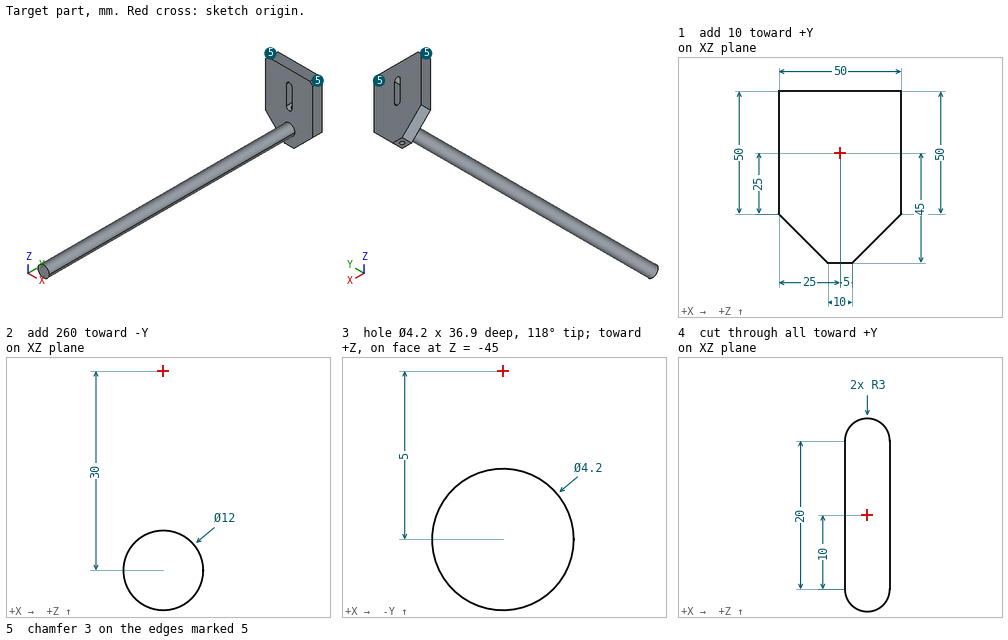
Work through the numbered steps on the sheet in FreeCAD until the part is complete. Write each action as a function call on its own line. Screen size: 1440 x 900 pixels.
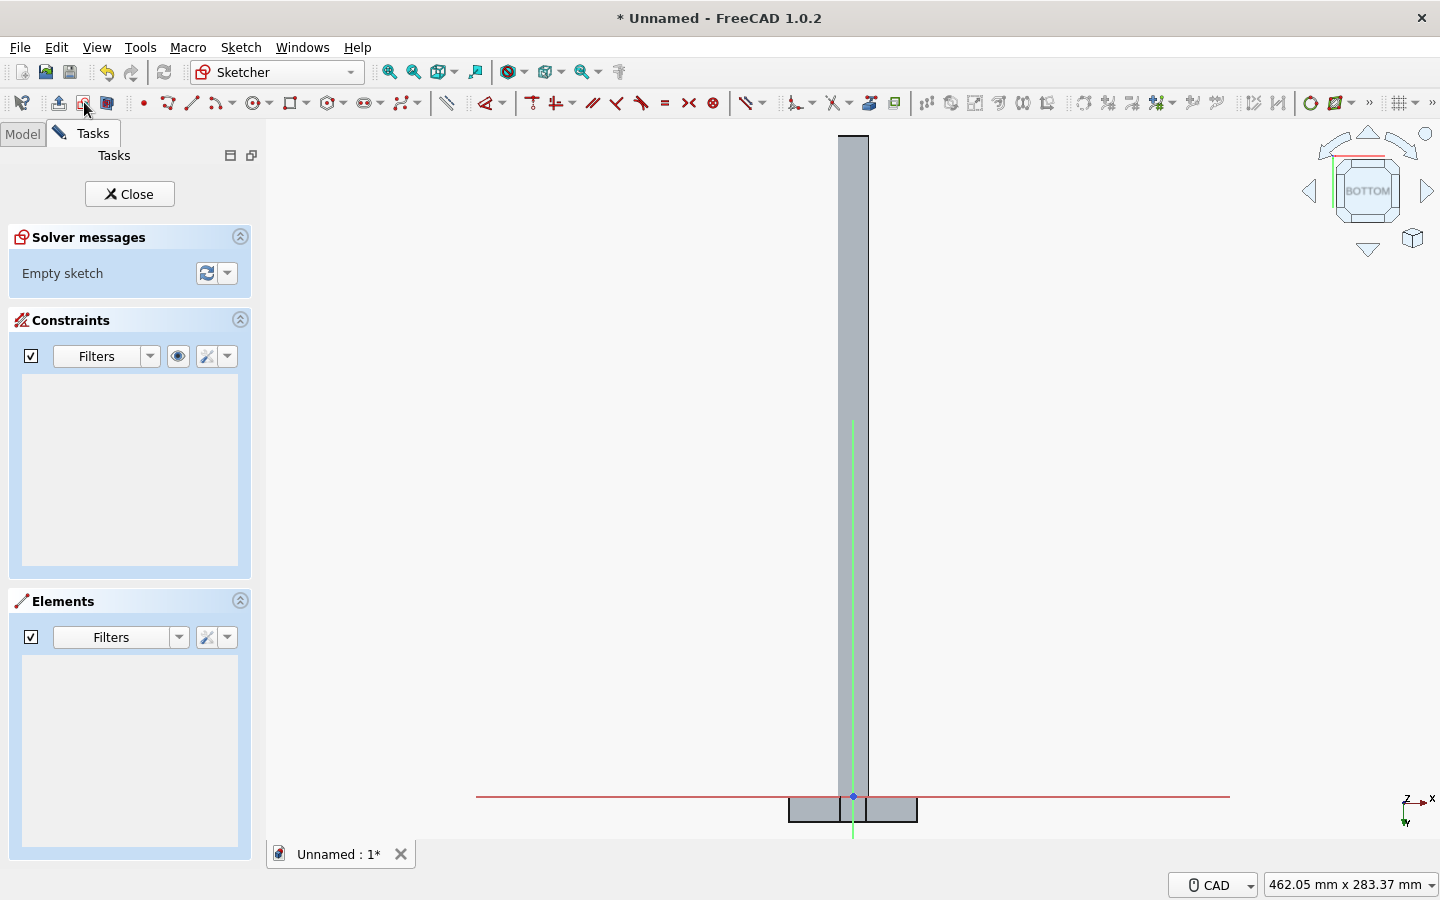
scroll(784, 479, down, 5)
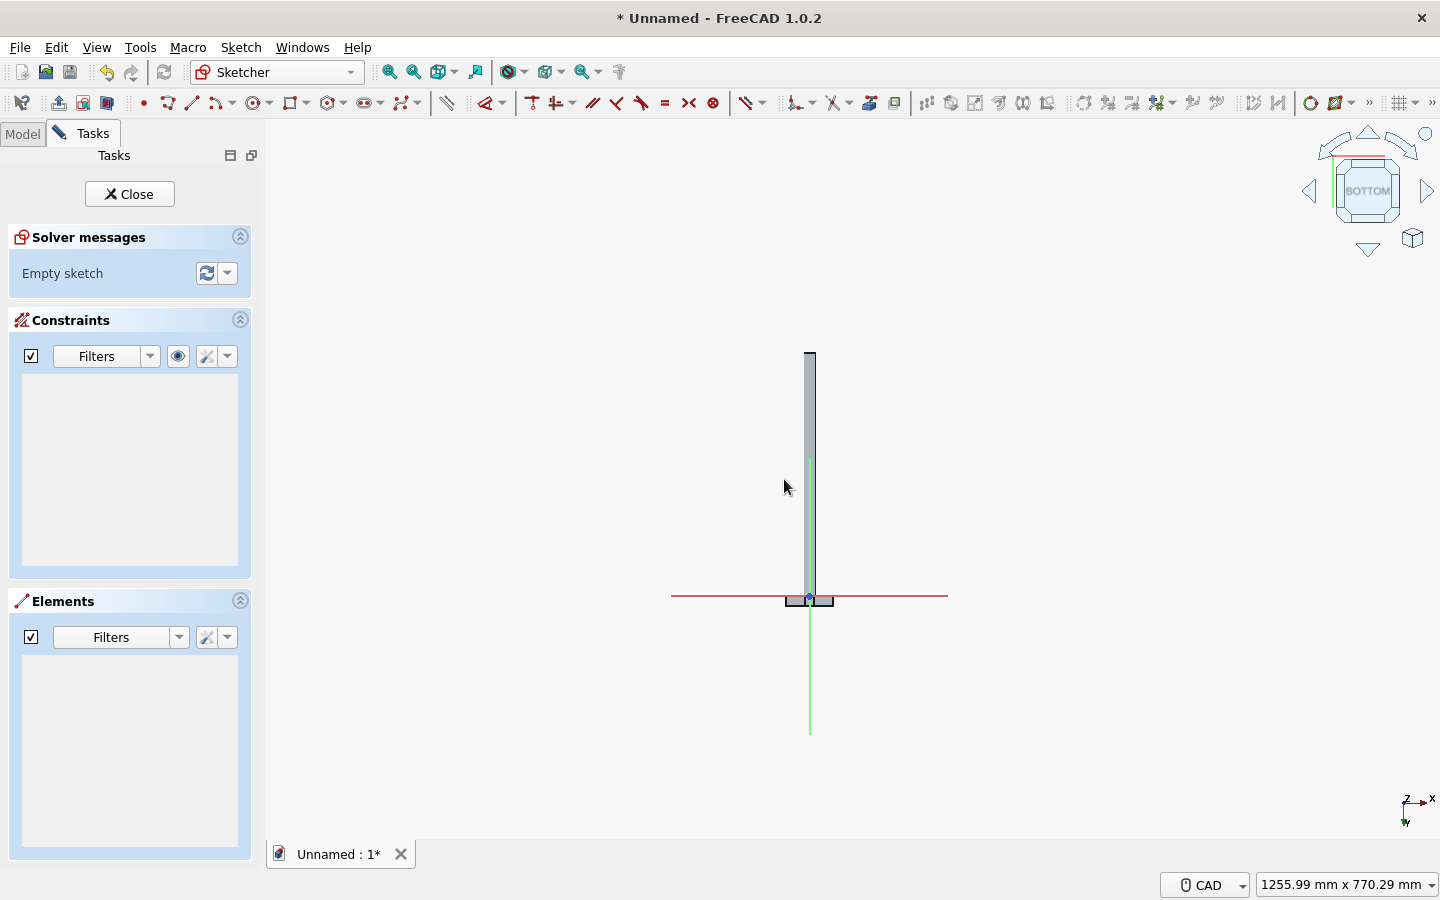
scroll(811, 606, up, 15)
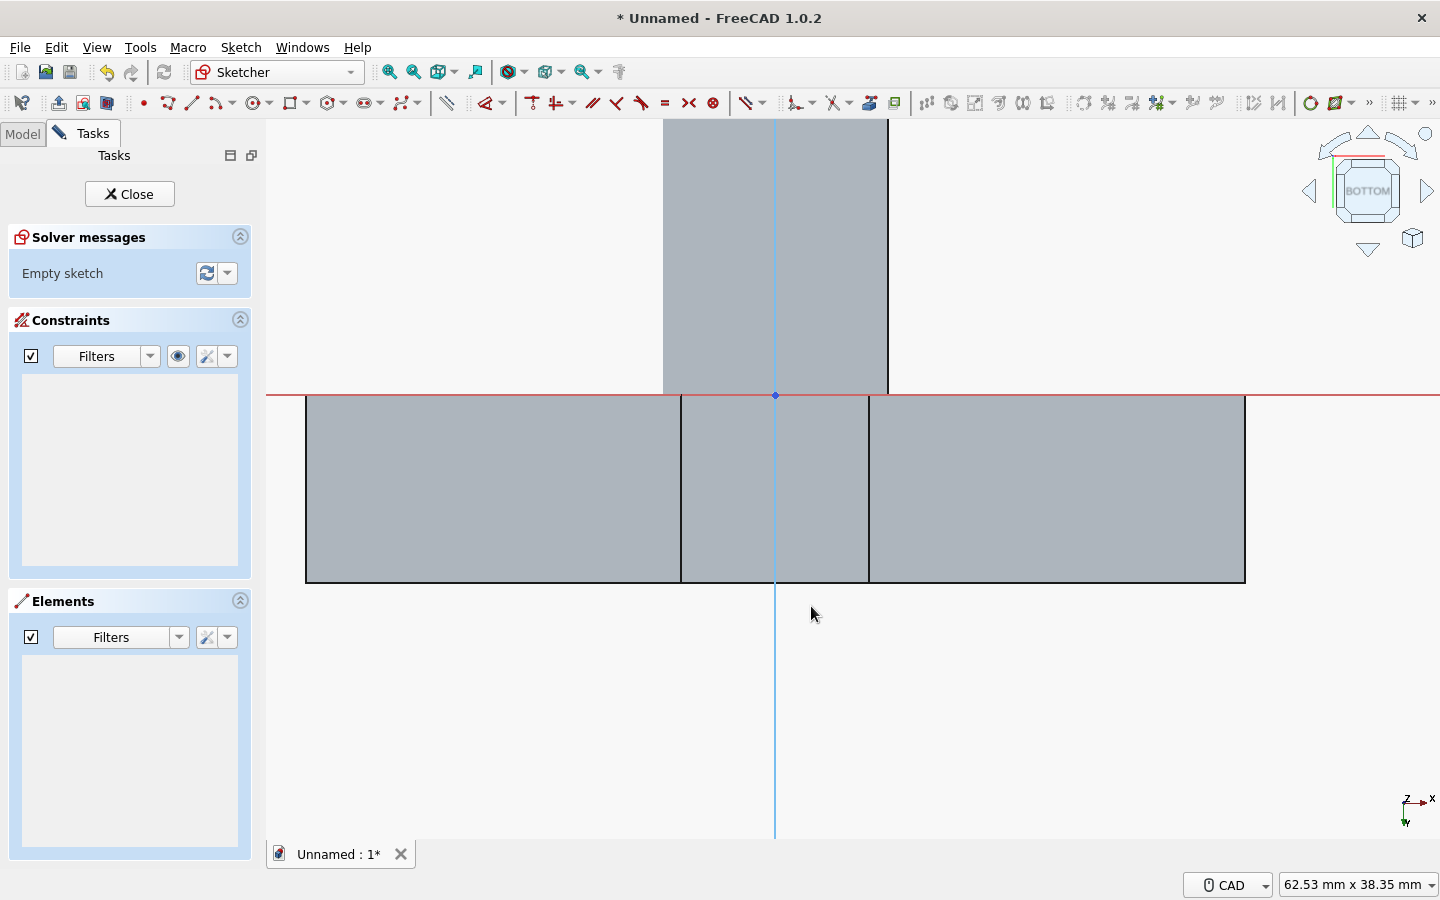
scroll(771, 455, up, 6)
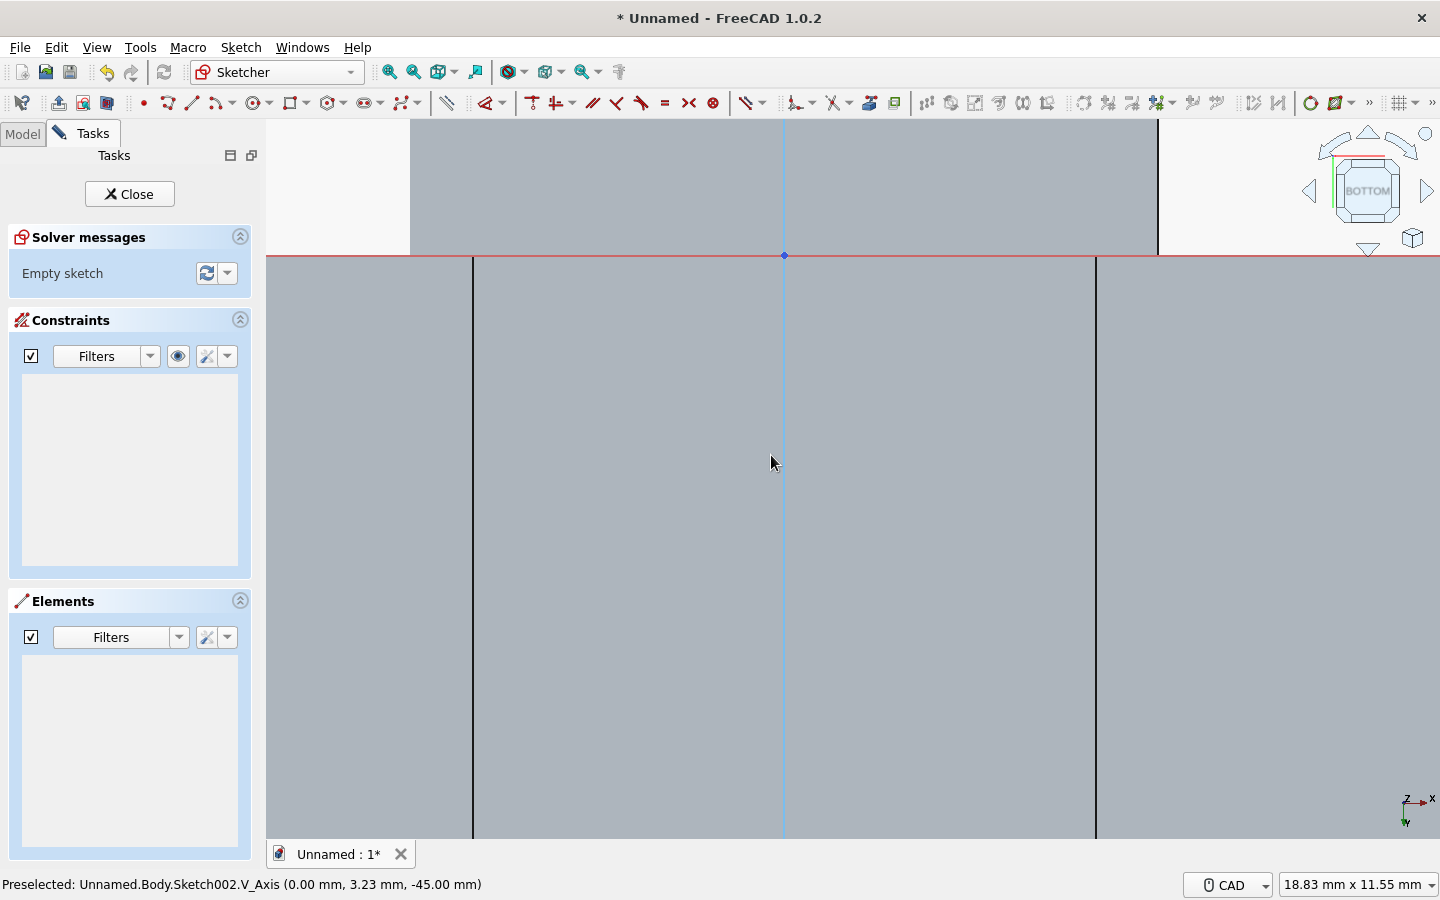
click(254, 104)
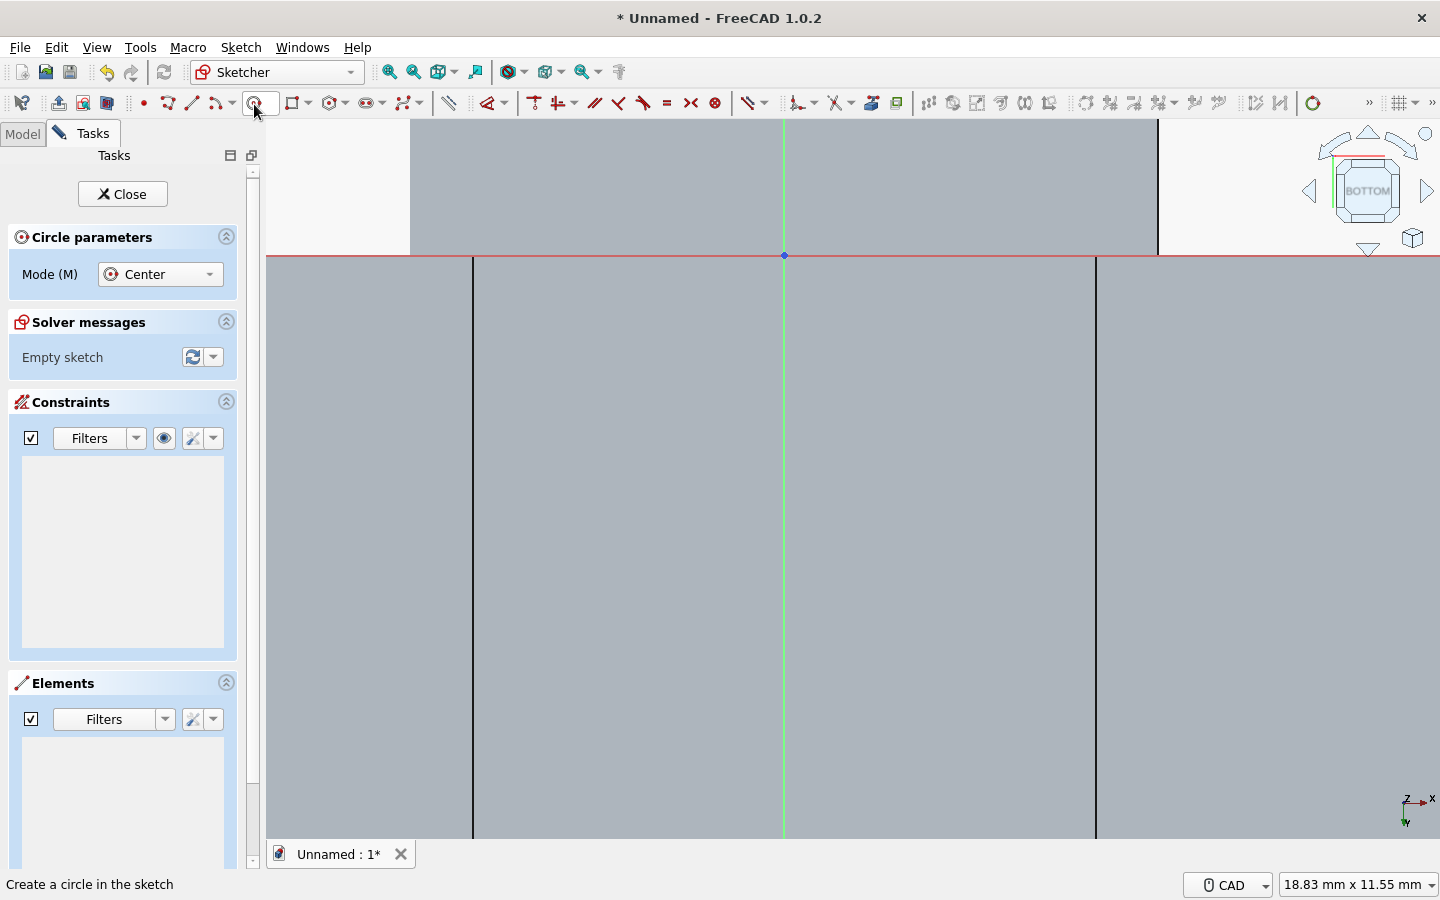
click(784, 568)
move(877, 475)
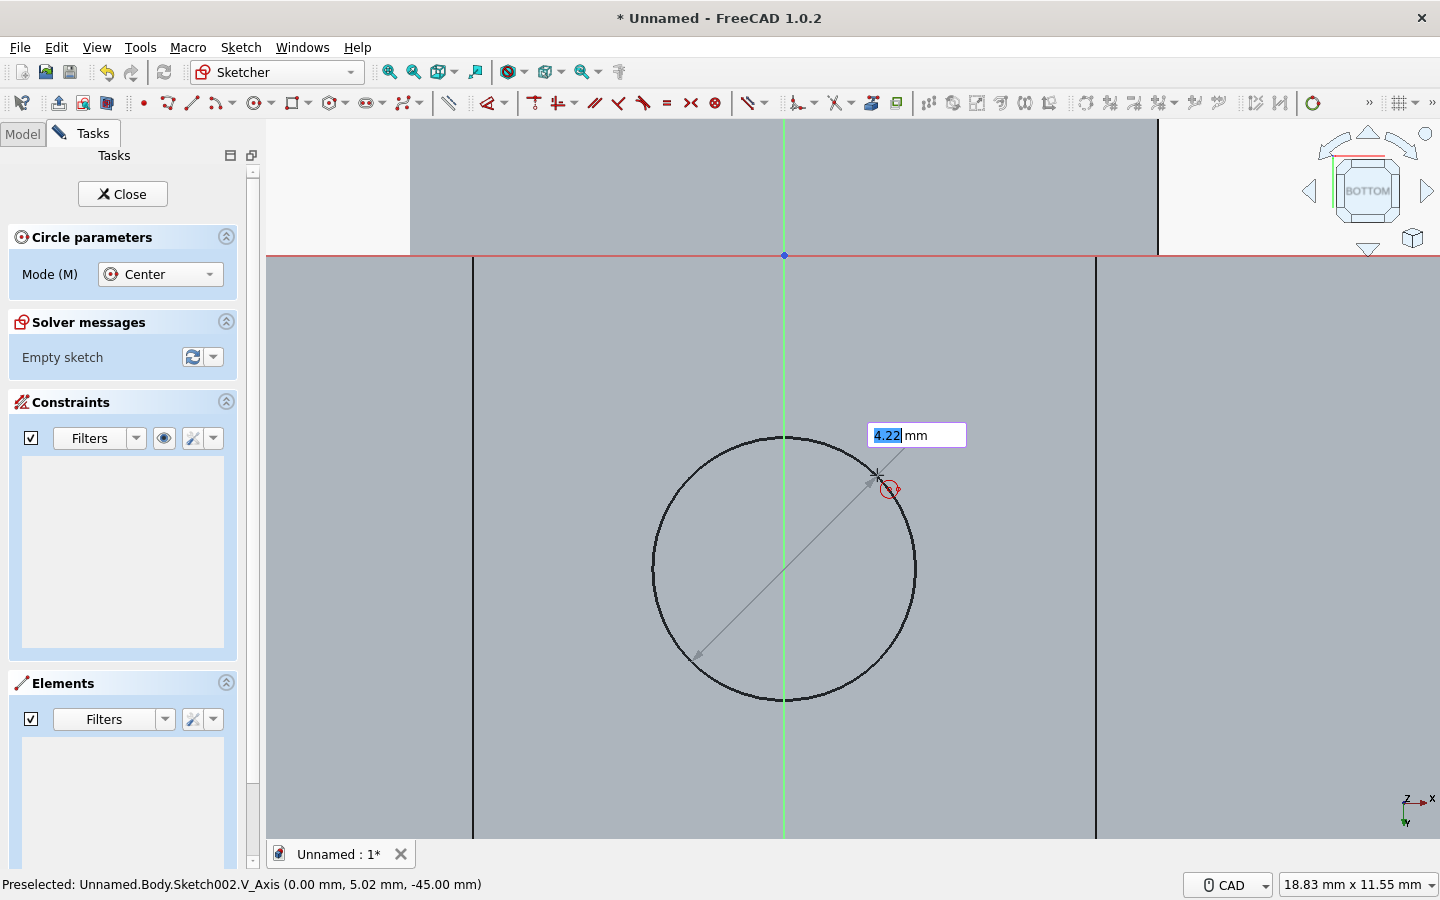
text(4.2)
key(Return)
key(Escape)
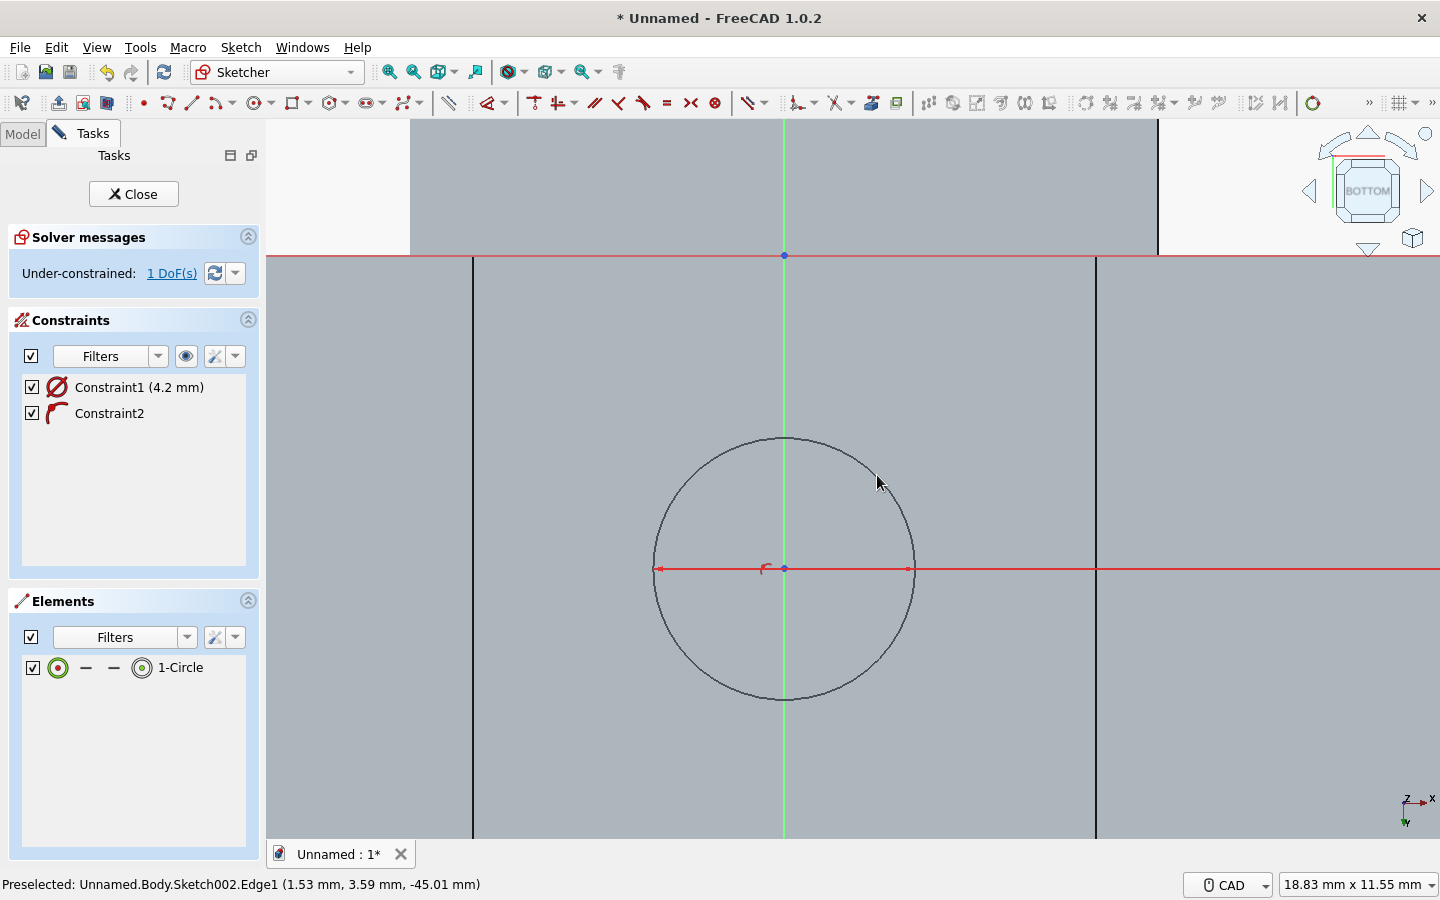
click(488, 104)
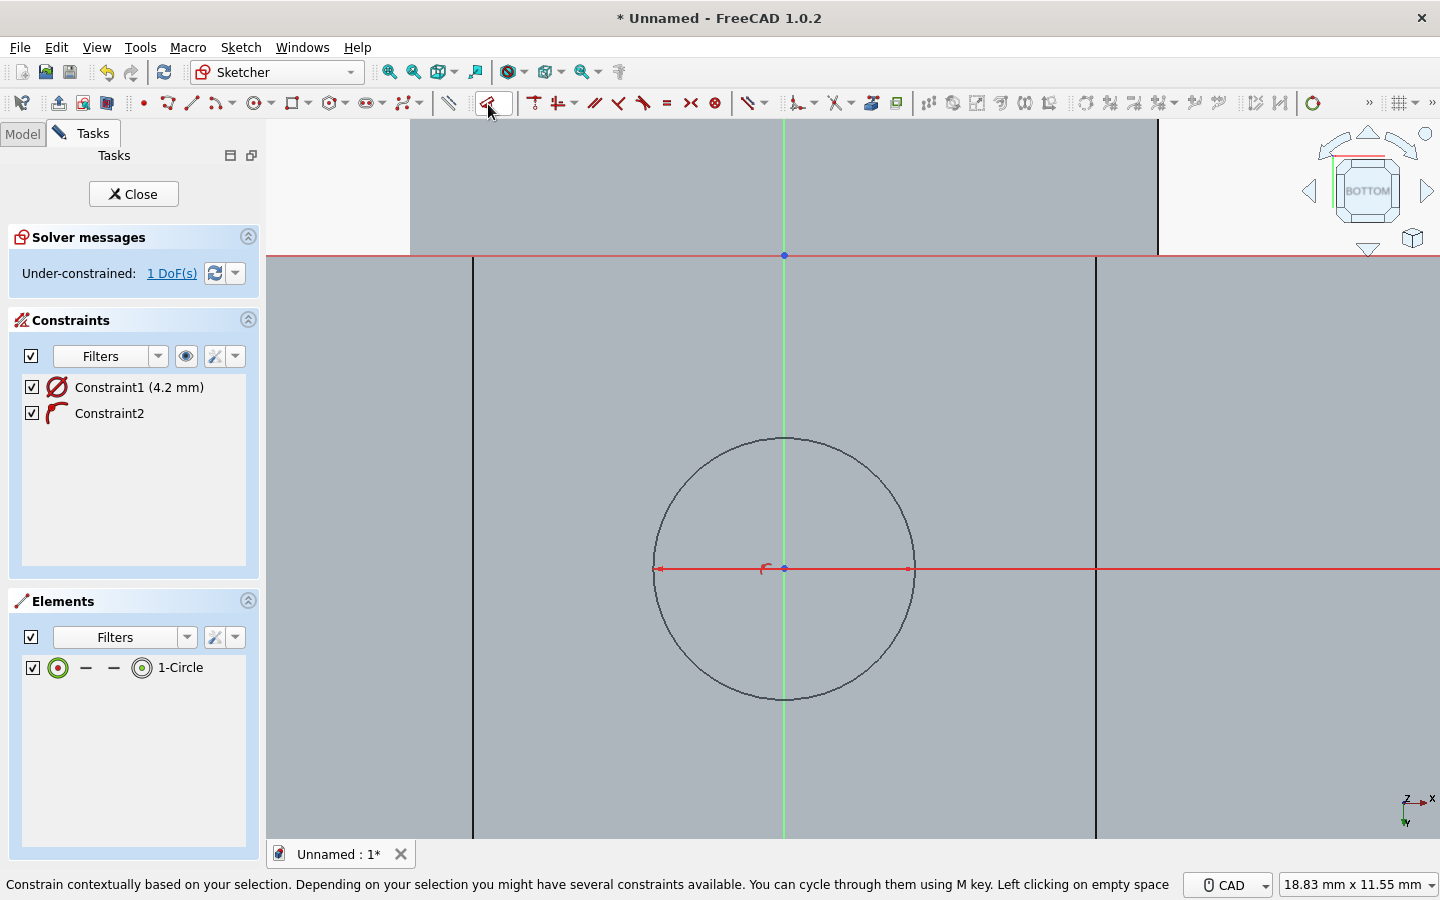
click(784, 569)
click(818, 412)